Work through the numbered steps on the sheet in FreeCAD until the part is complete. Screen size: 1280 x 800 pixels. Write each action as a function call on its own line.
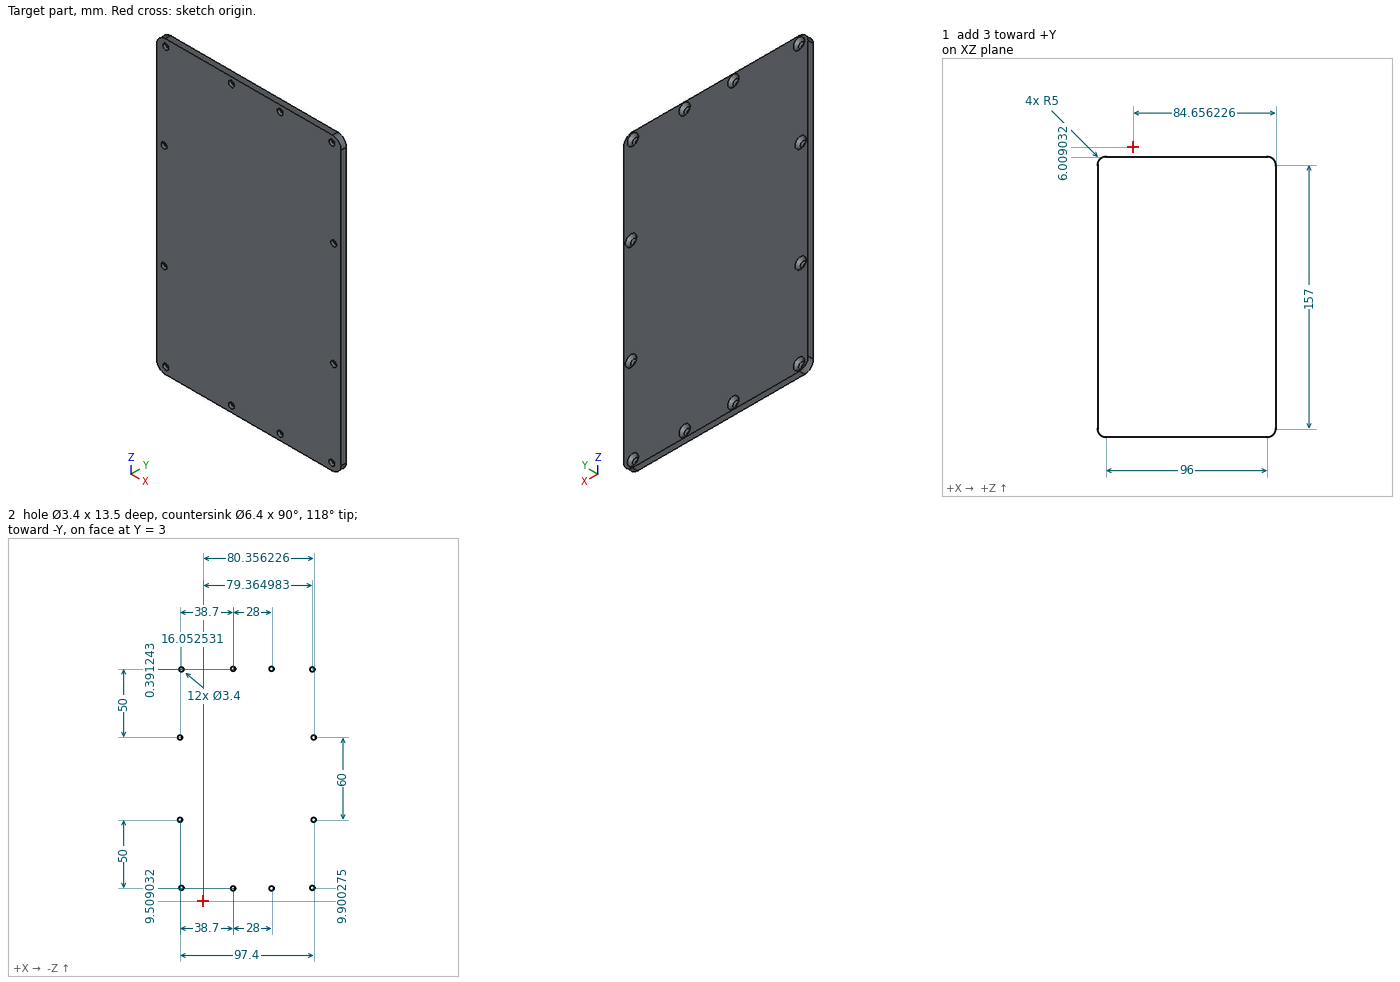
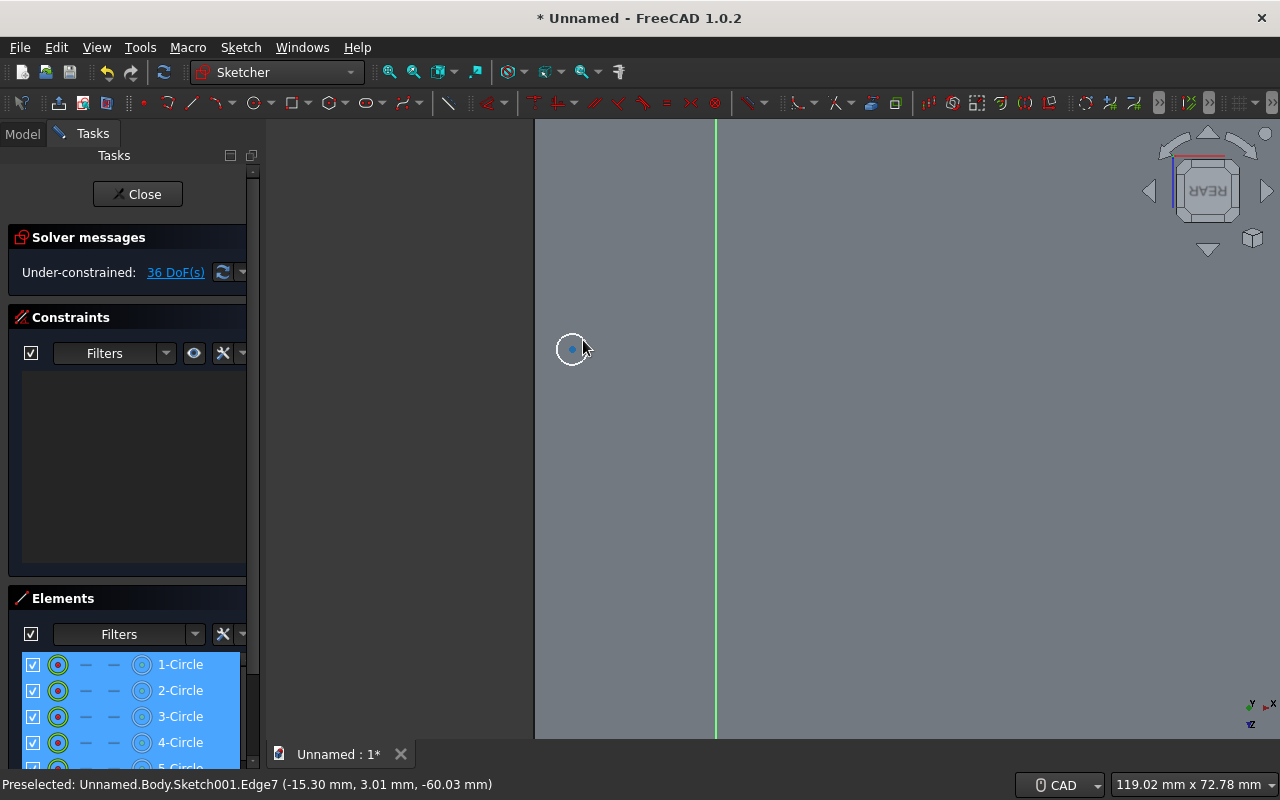
click(583, 339)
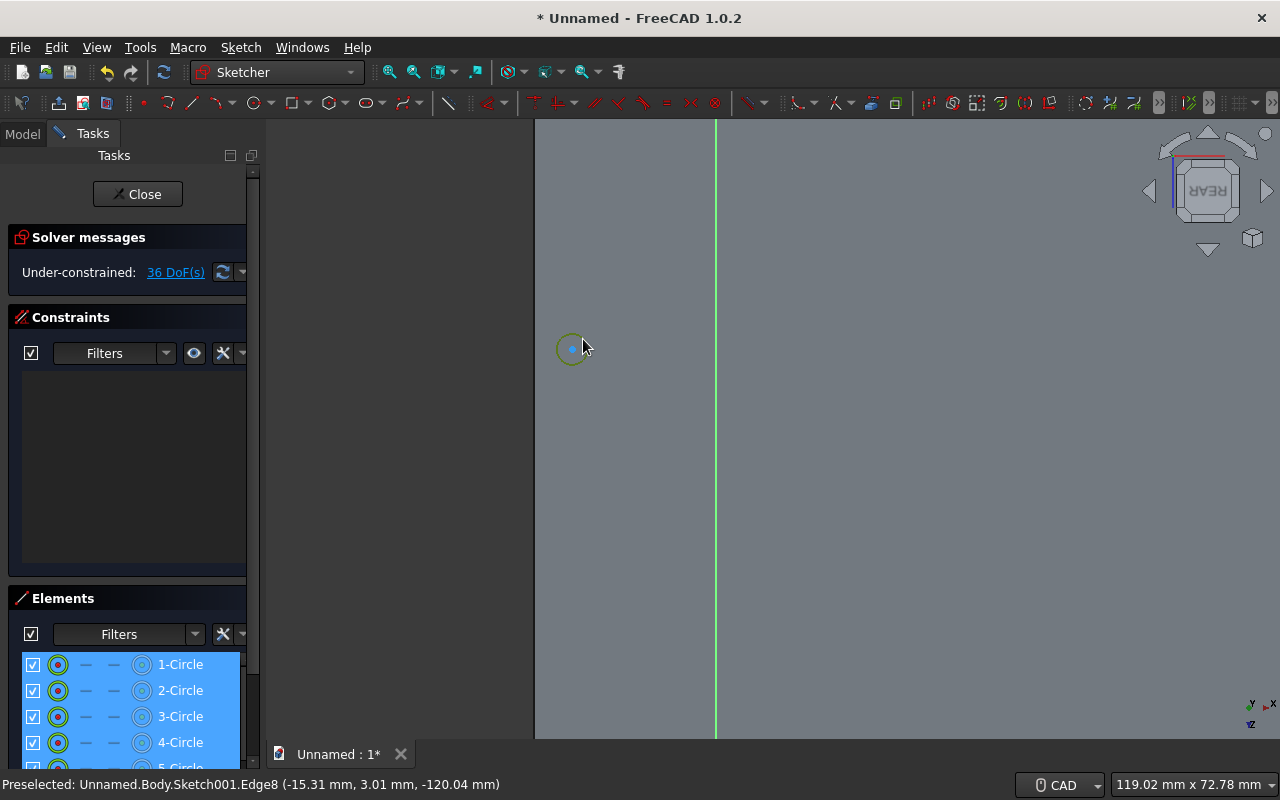
scroll(583, 340, down, 6)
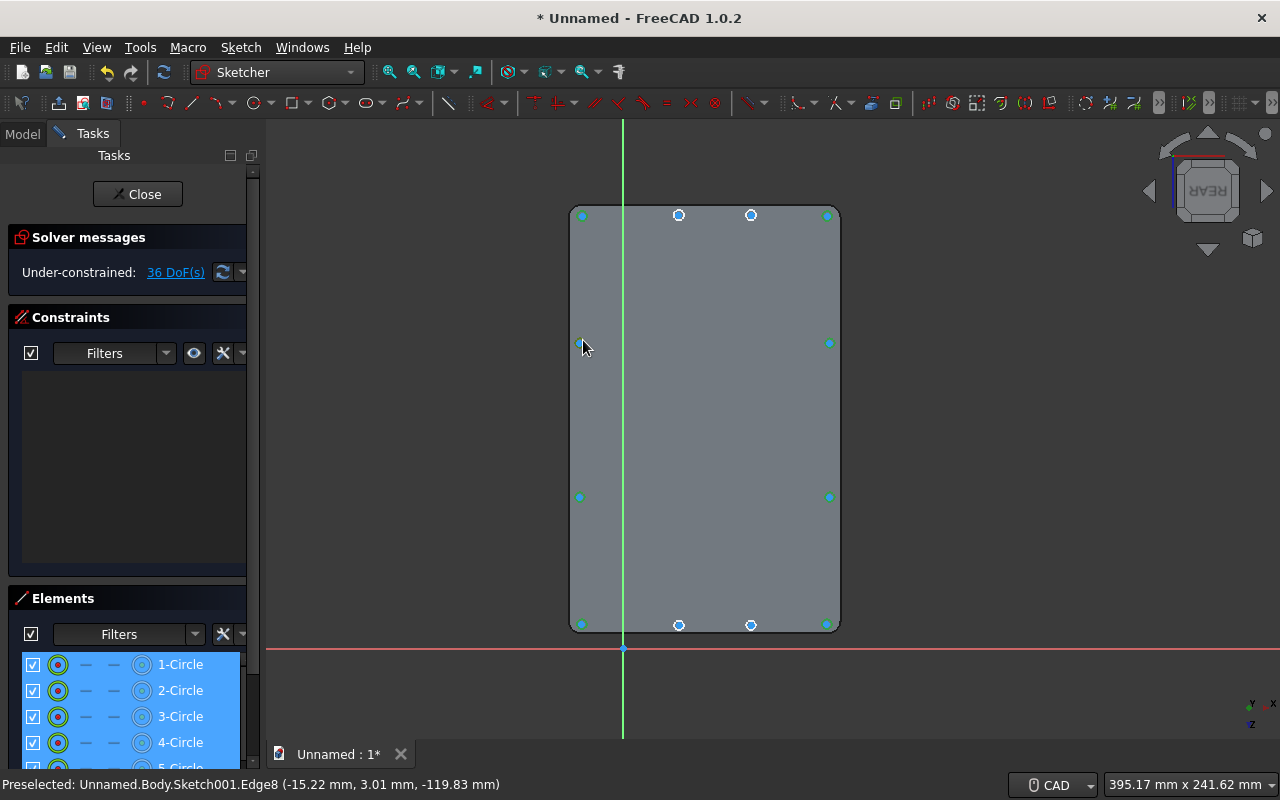
scroll(683, 211, up, 5)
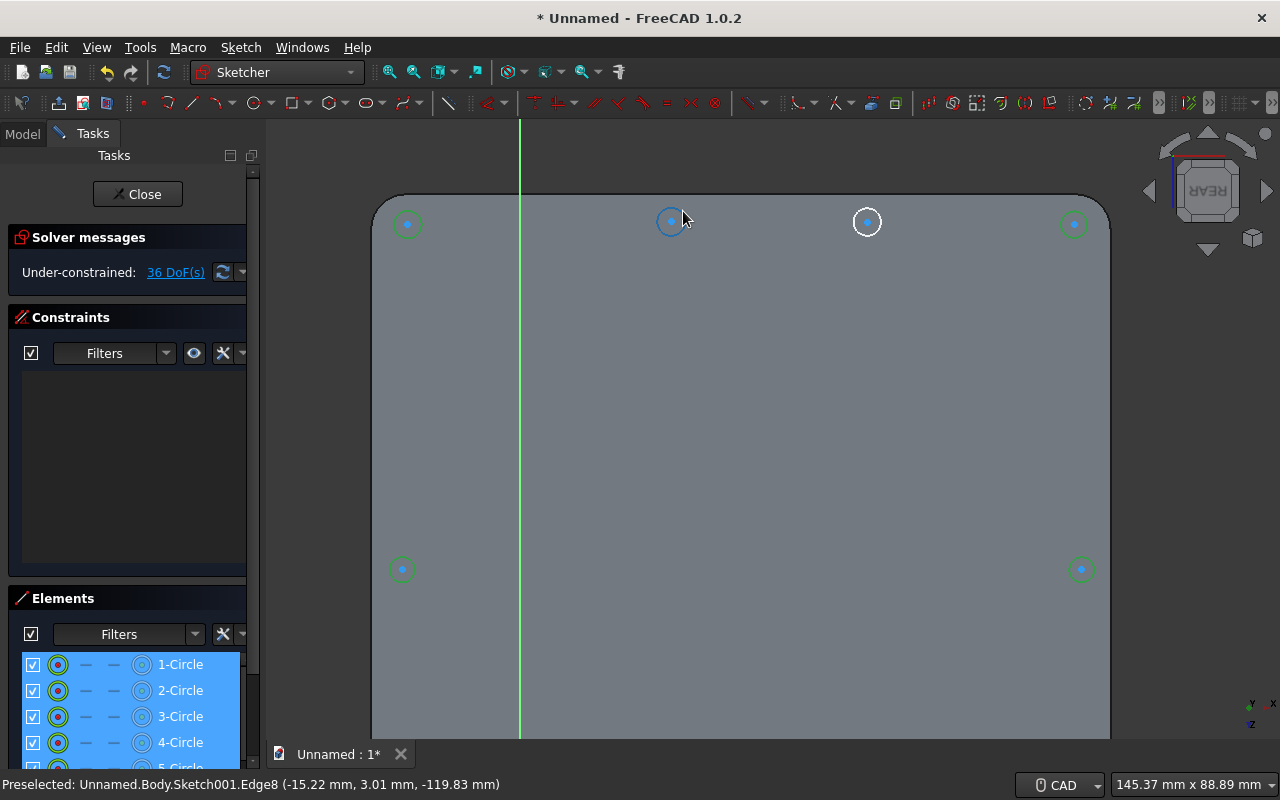
click(681, 212)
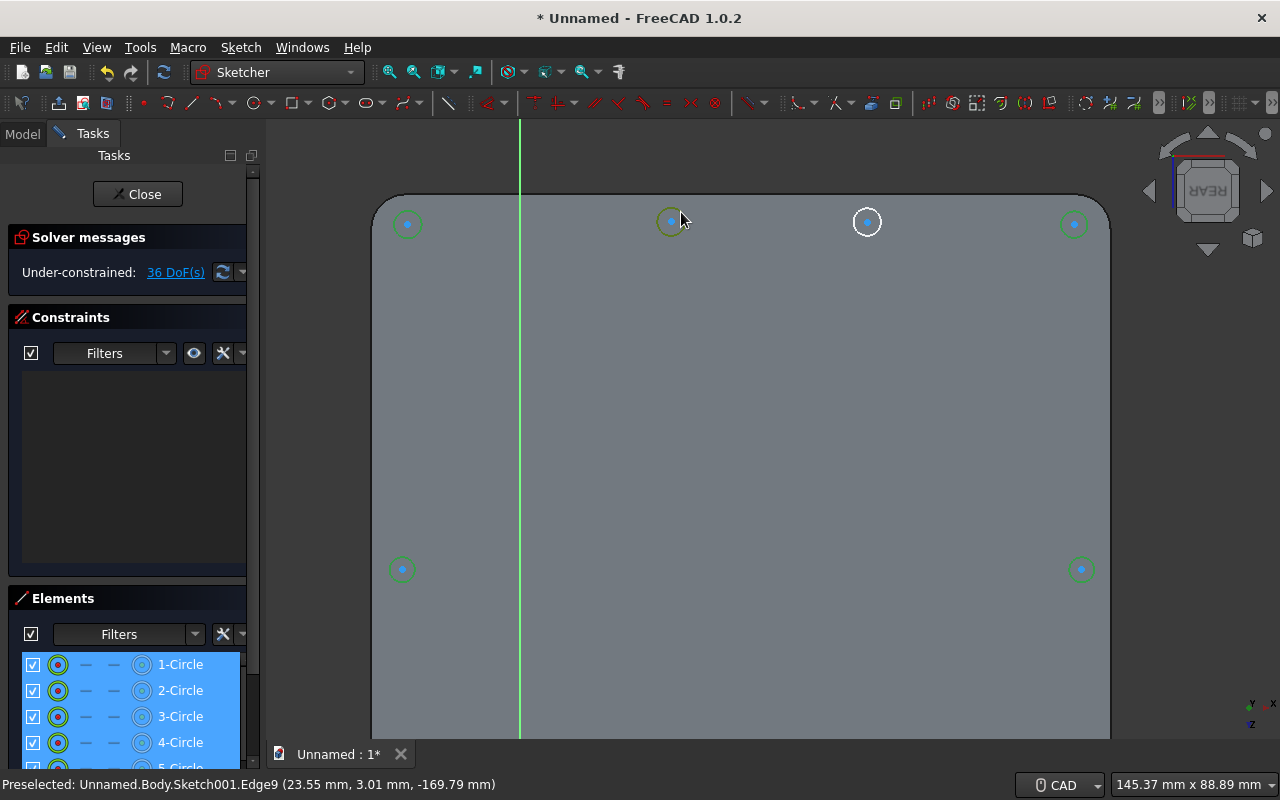
click(877, 212)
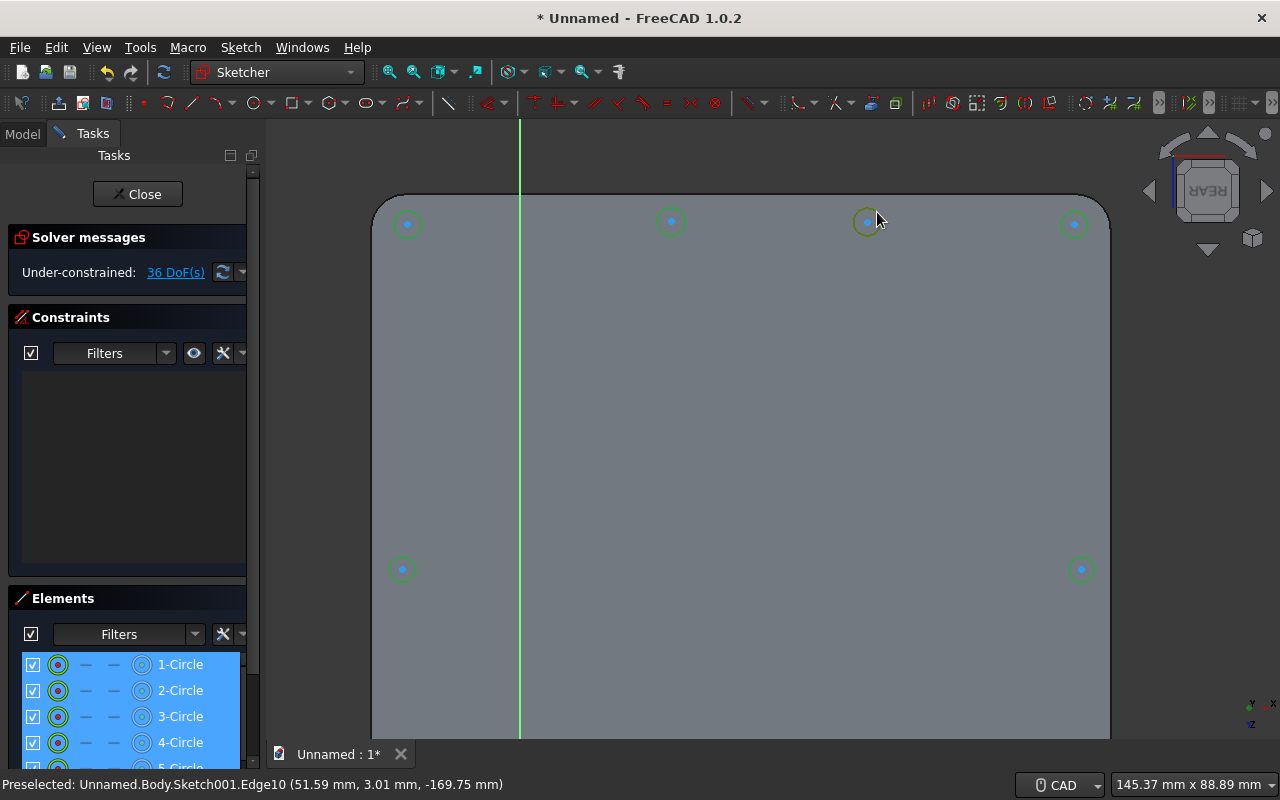
scroll(683, 211, down, 5)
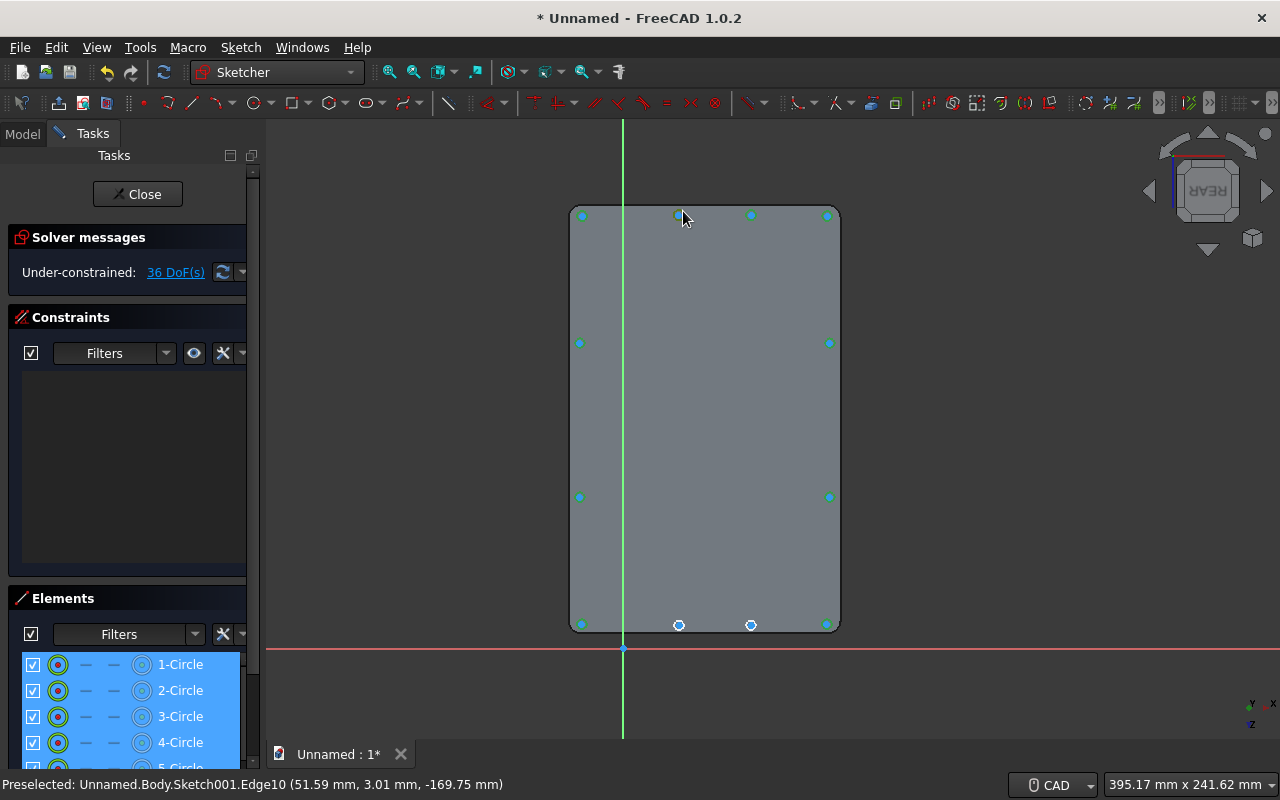
scroll(682, 622, up, 6)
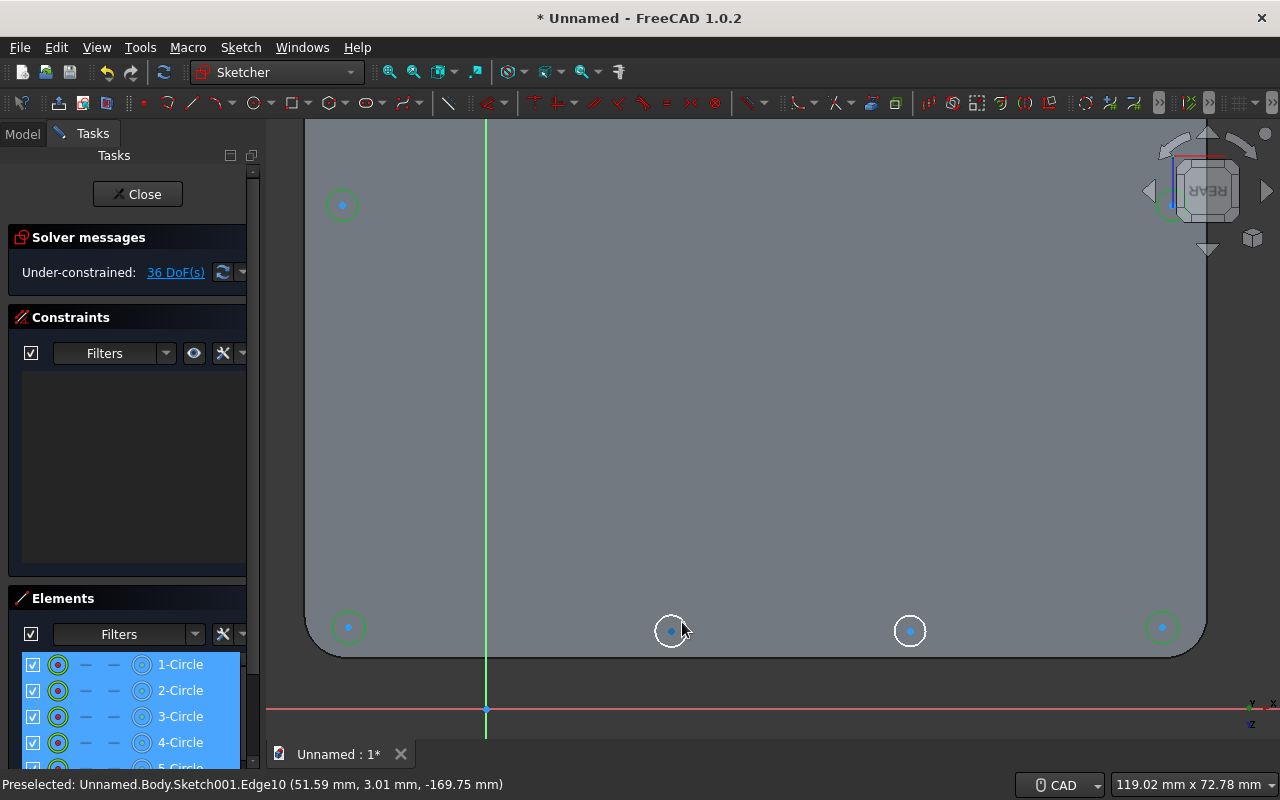
click(682, 620)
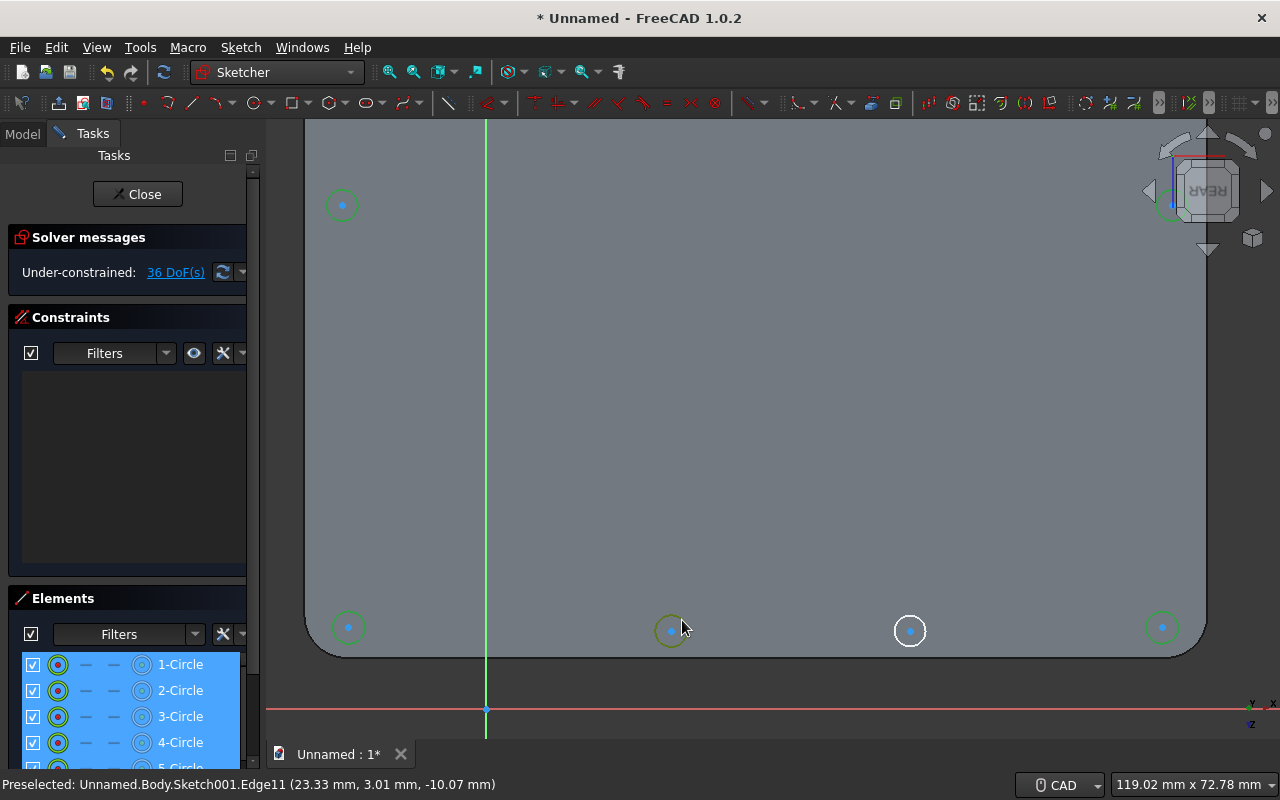
click(921, 620)